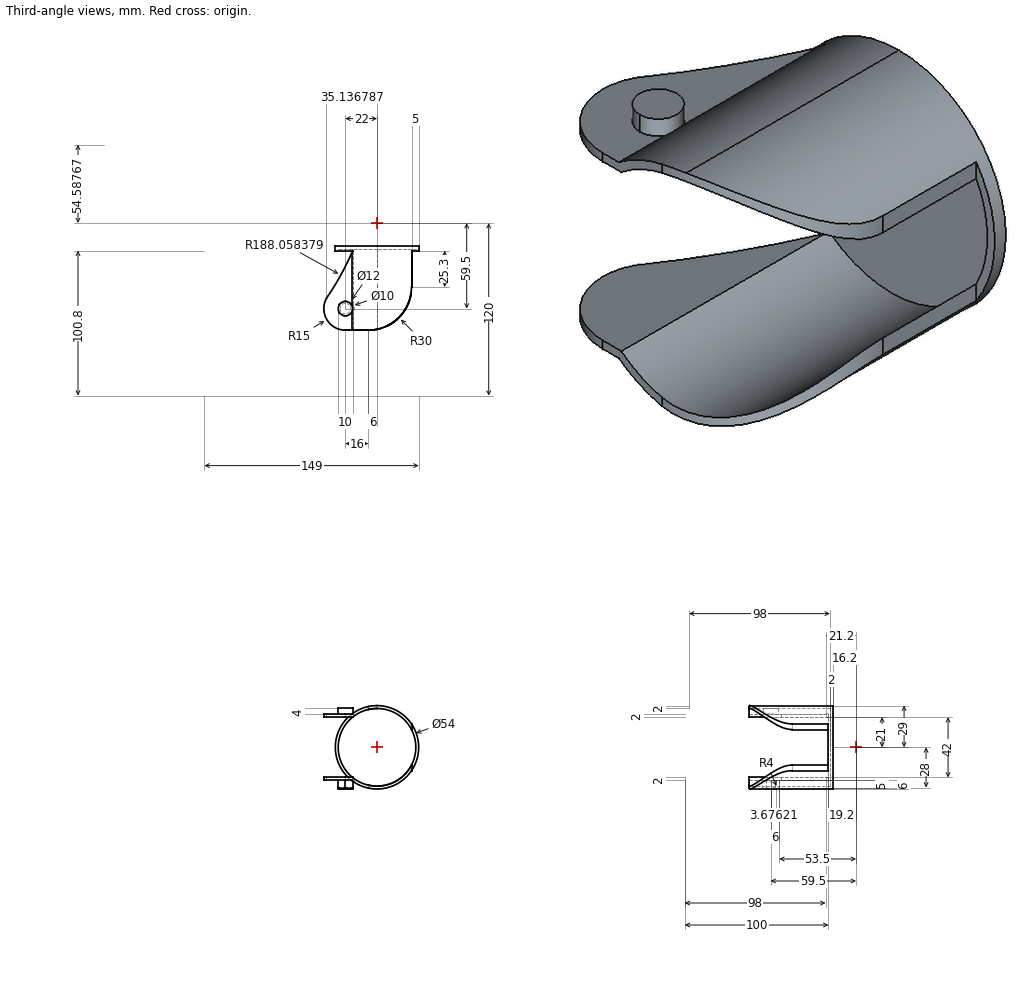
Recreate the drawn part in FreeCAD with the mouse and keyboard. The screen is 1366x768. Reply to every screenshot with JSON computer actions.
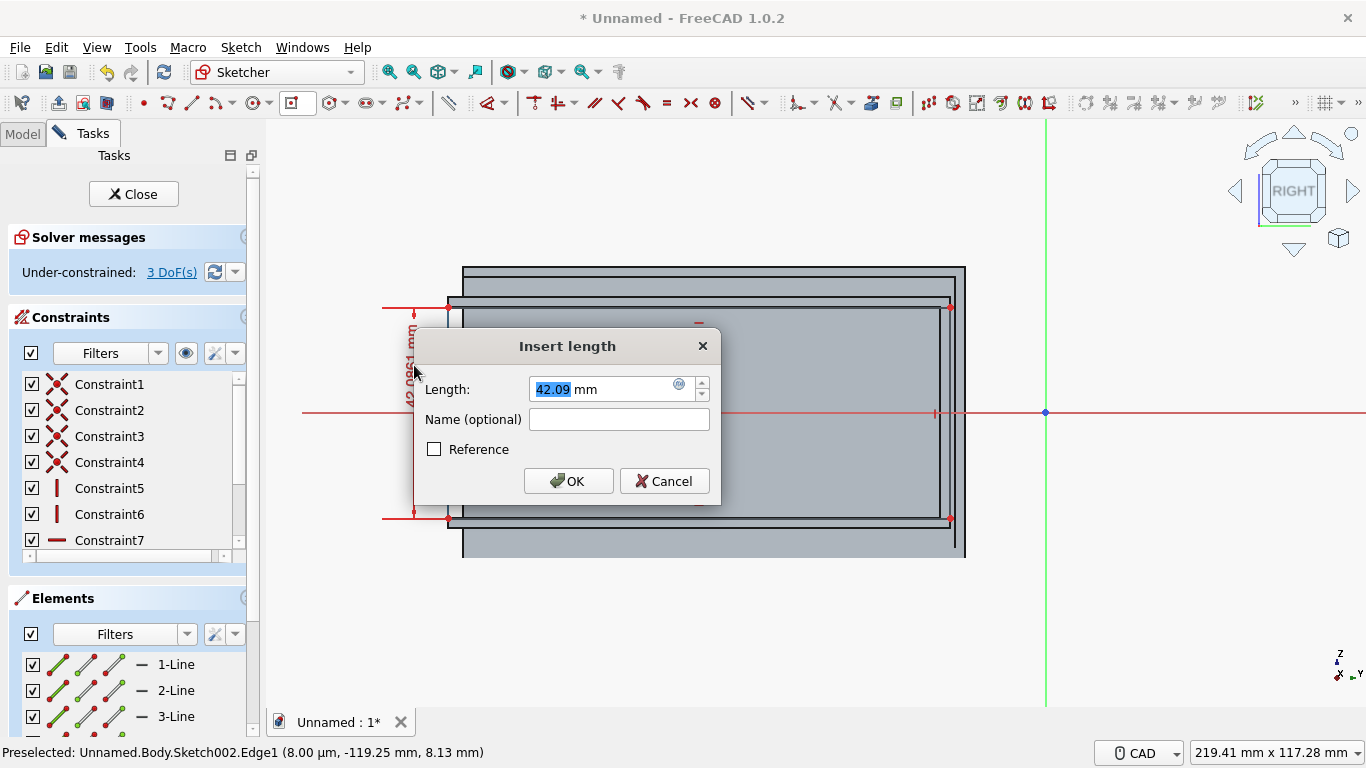
{"action": "type", "text": "42"}
{"action": "key", "text": "Return"}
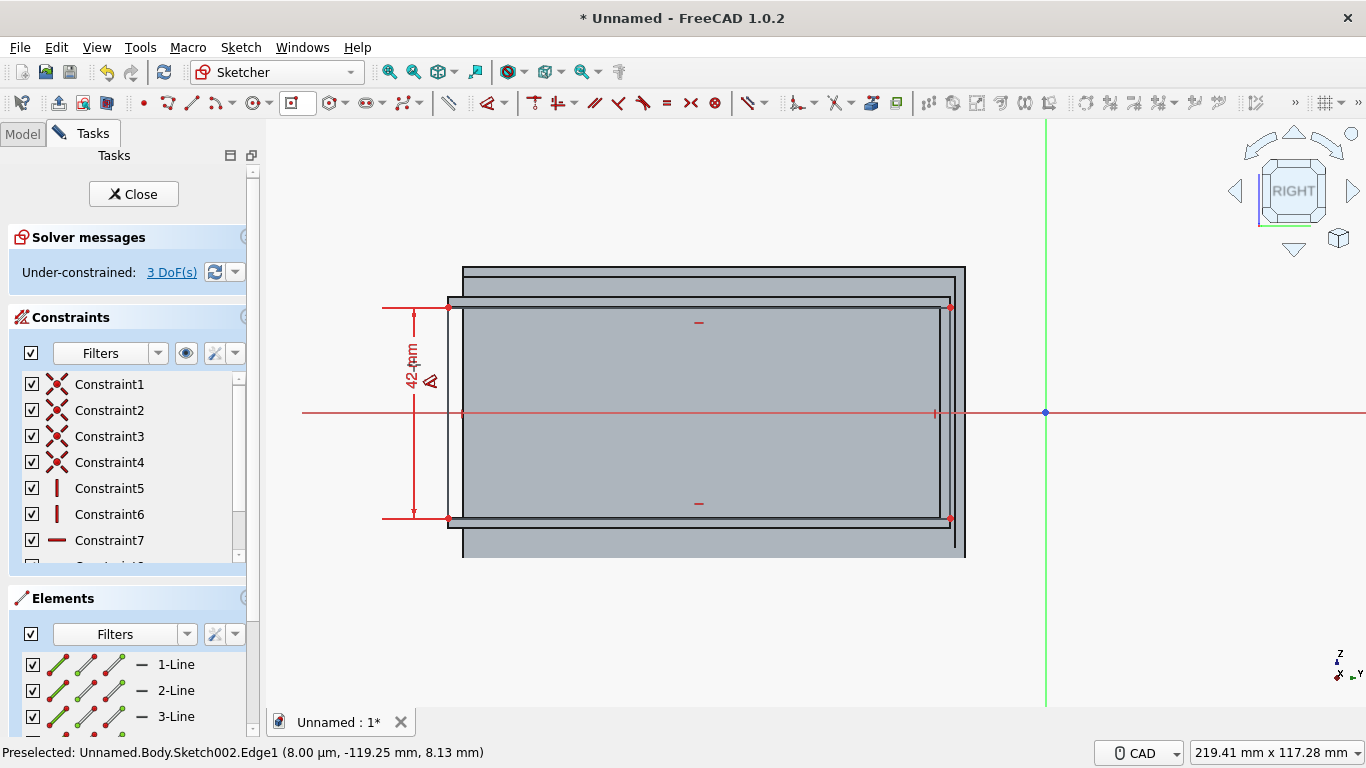
{"action": "left_click", "coordinate": [599, 519]}
{"action": "left_click", "coordinate": [699, 553]}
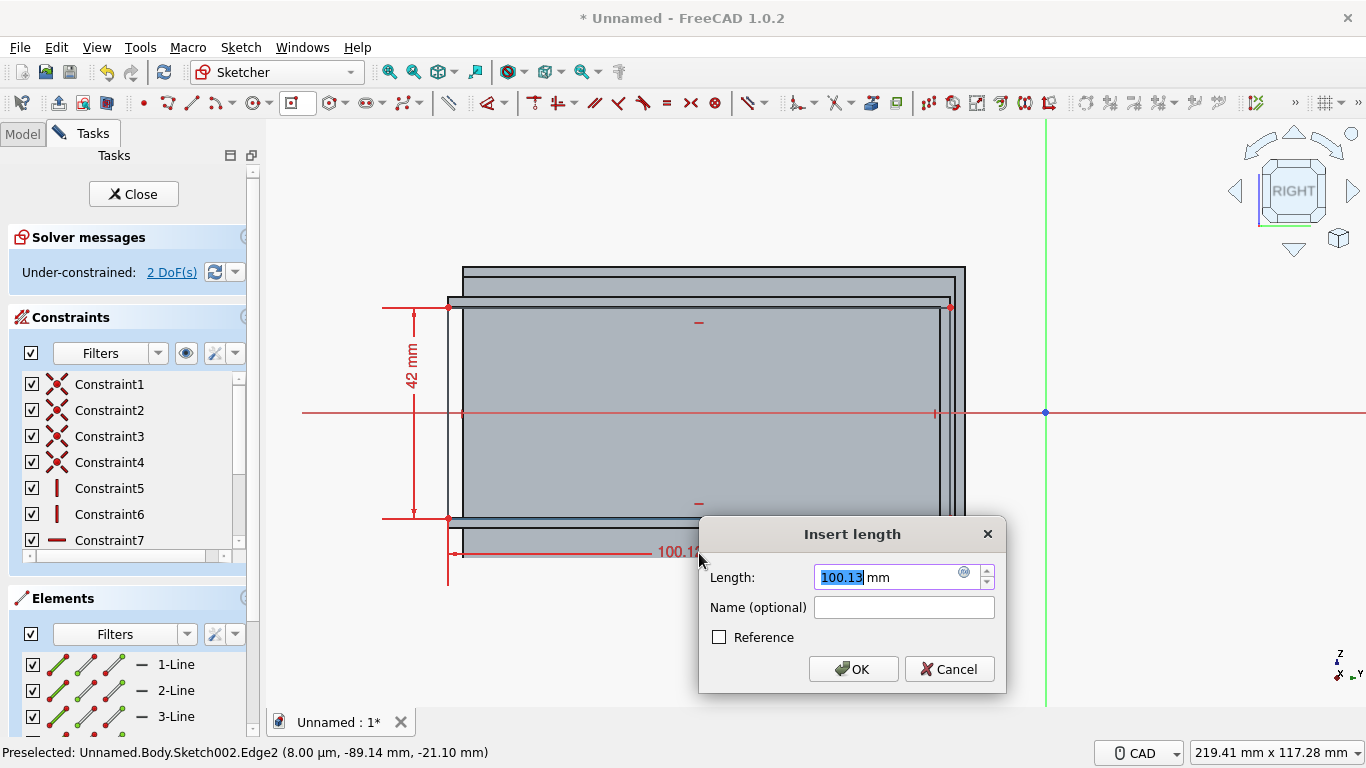
{"action": "type", "text": "100"}
{"action": "key", "text": "Return"}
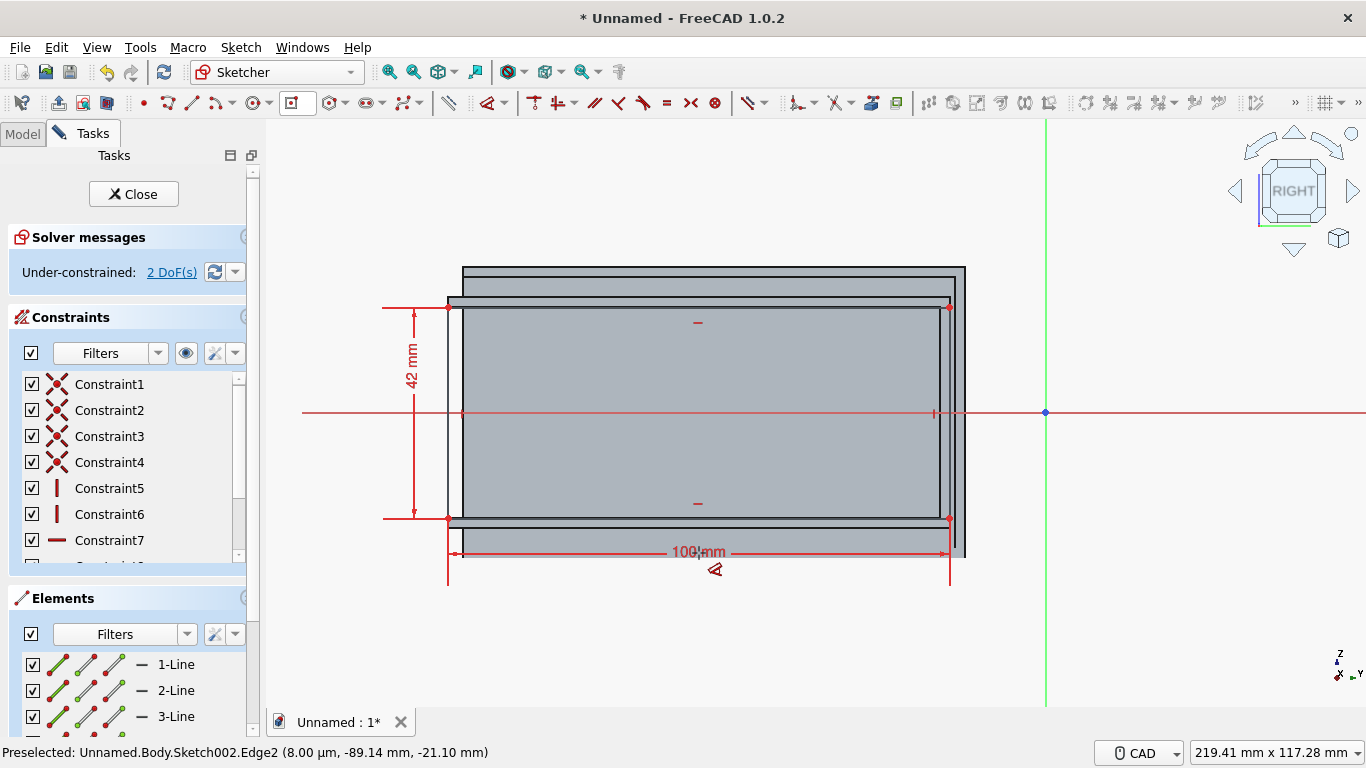
{"action": "left_click", "coordinate": [448, 308]}
{"action": "left_click", "coordinate": [414, 336]}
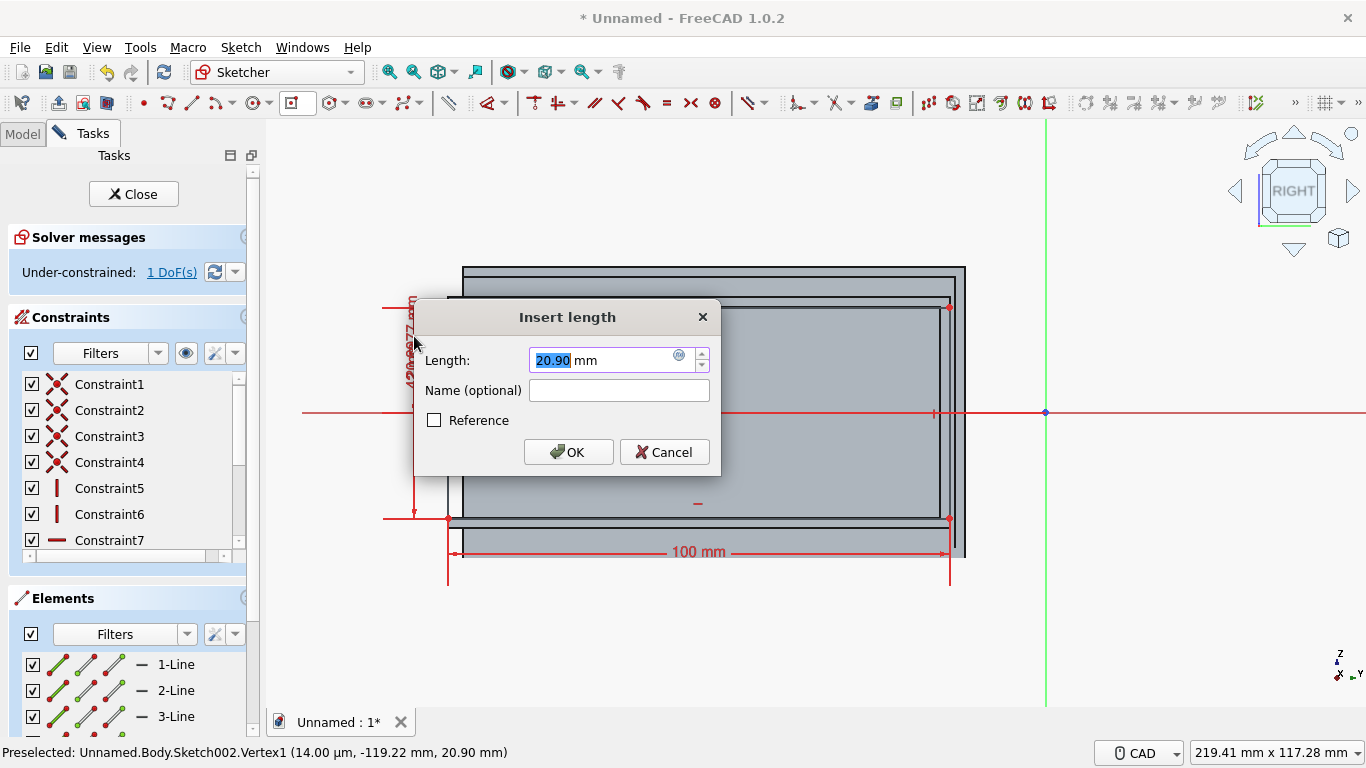
{"action": "type", "text": "21"}
{"action": "key", "text": "Return"}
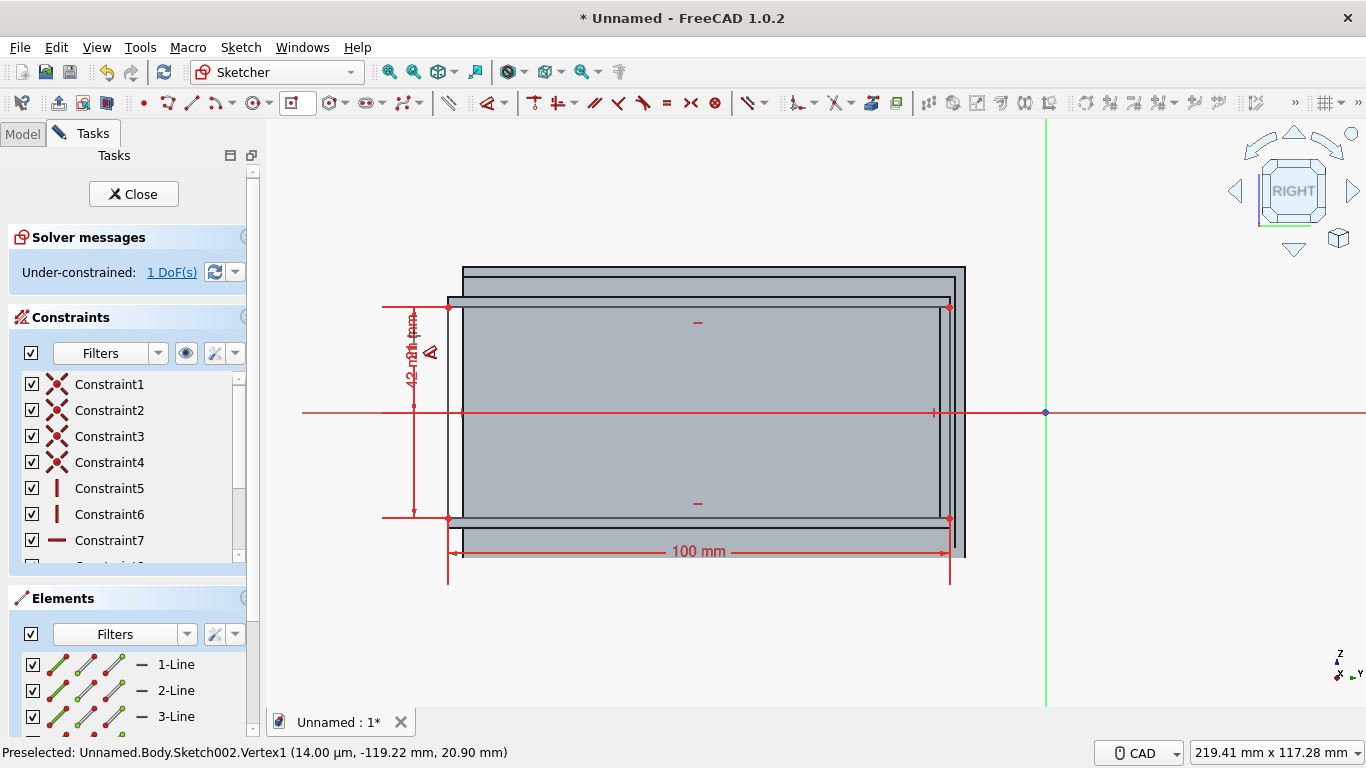
{"action": "left_click", "coordinate": [950, 518]}
{"action": "left_click", "coordinate": [998, 552]}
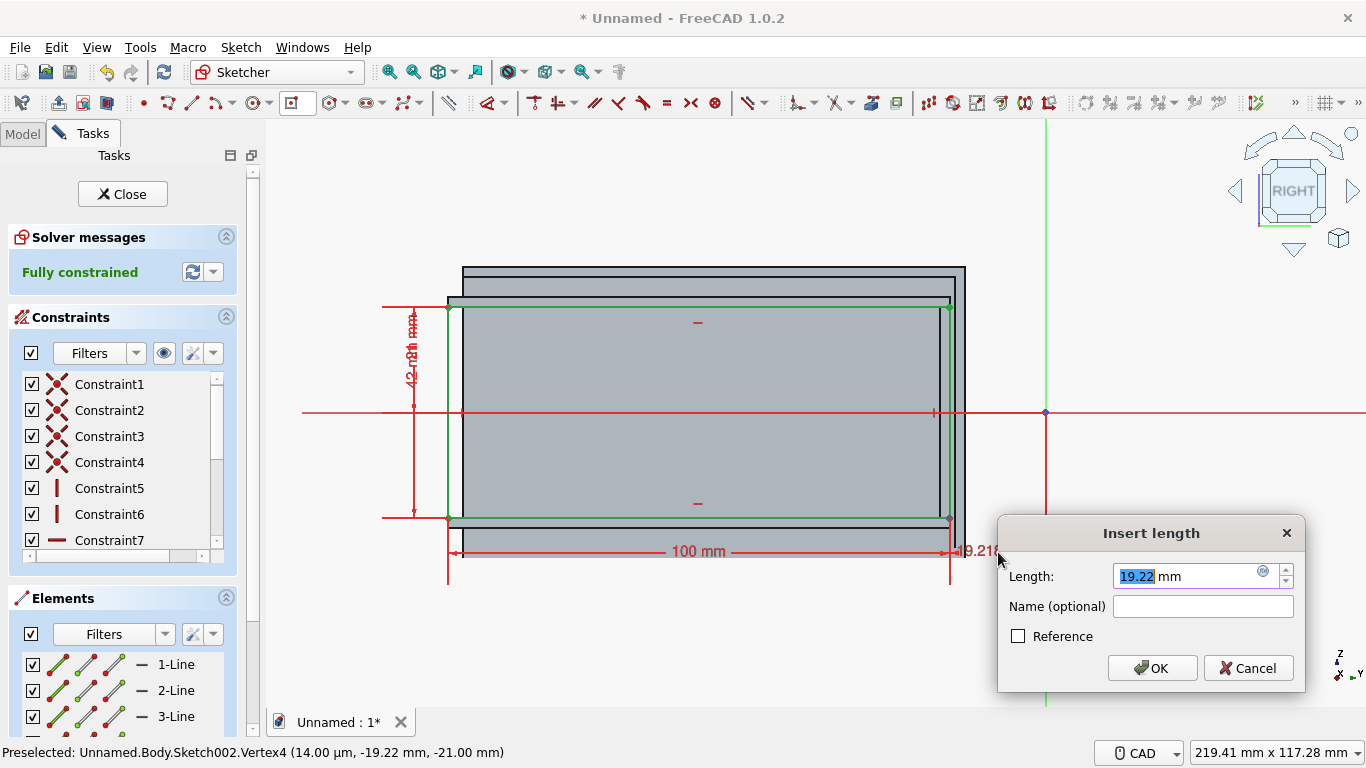
{"action": "type", "text": "19.2"}
{"action": "key", "text": "Return"}
{"action": "key", "text": "Escape"}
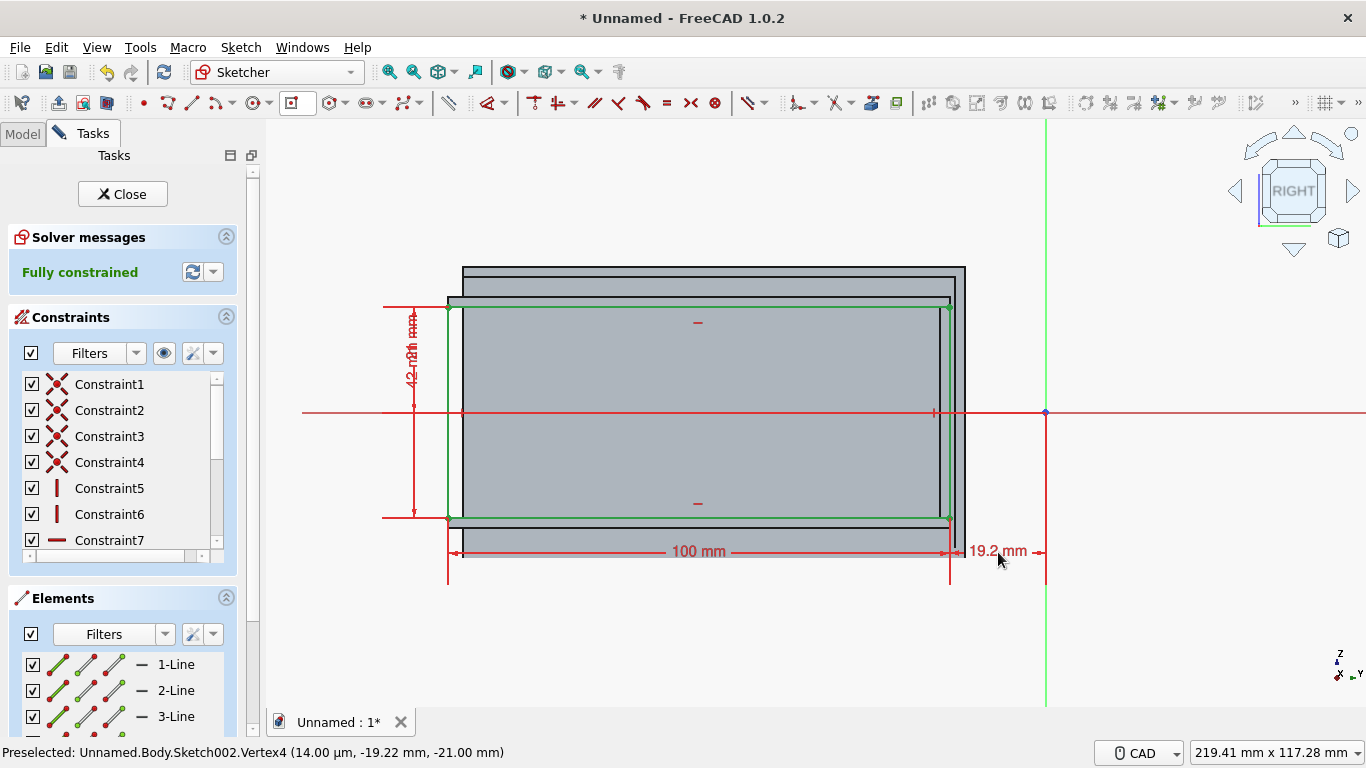
{"action": "left_click", "coordinate": [123, 194]}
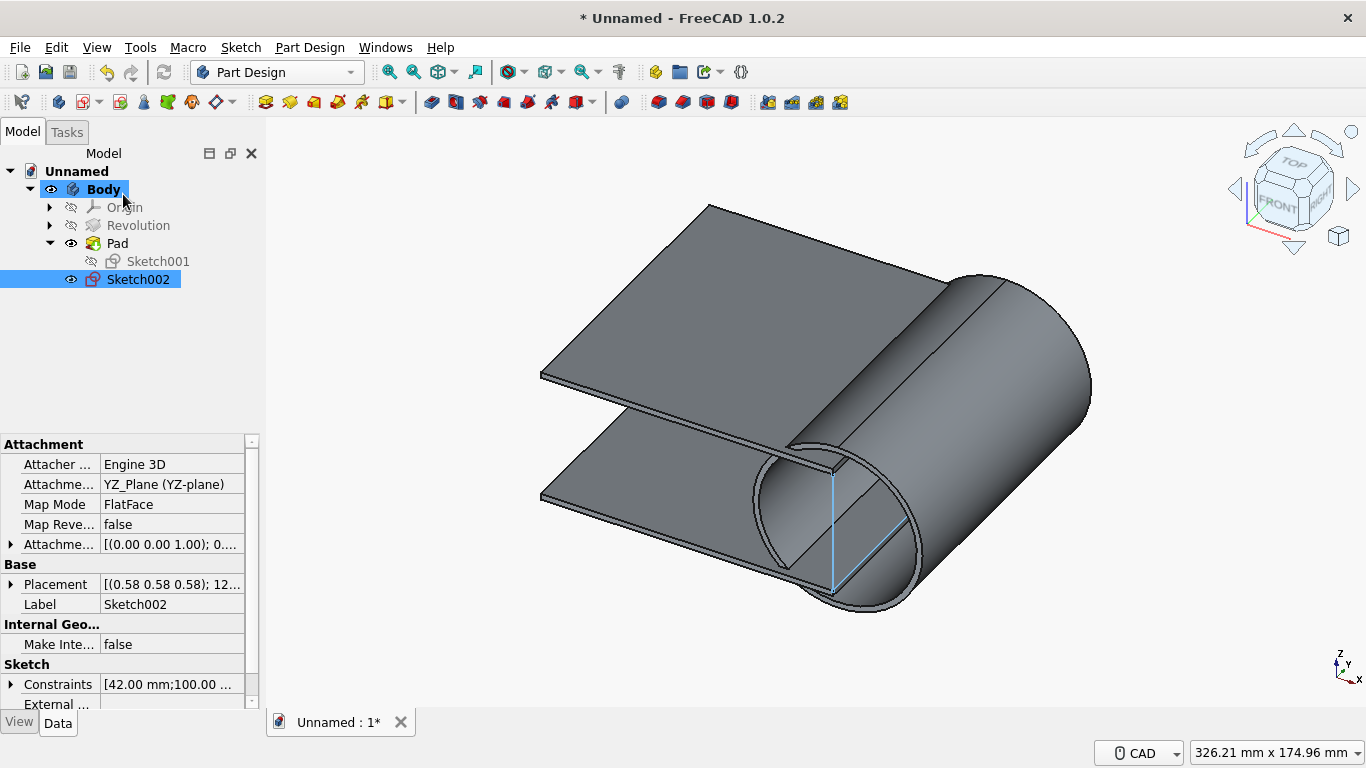
{"action": "left_click", "coordinate": [432, 102]}